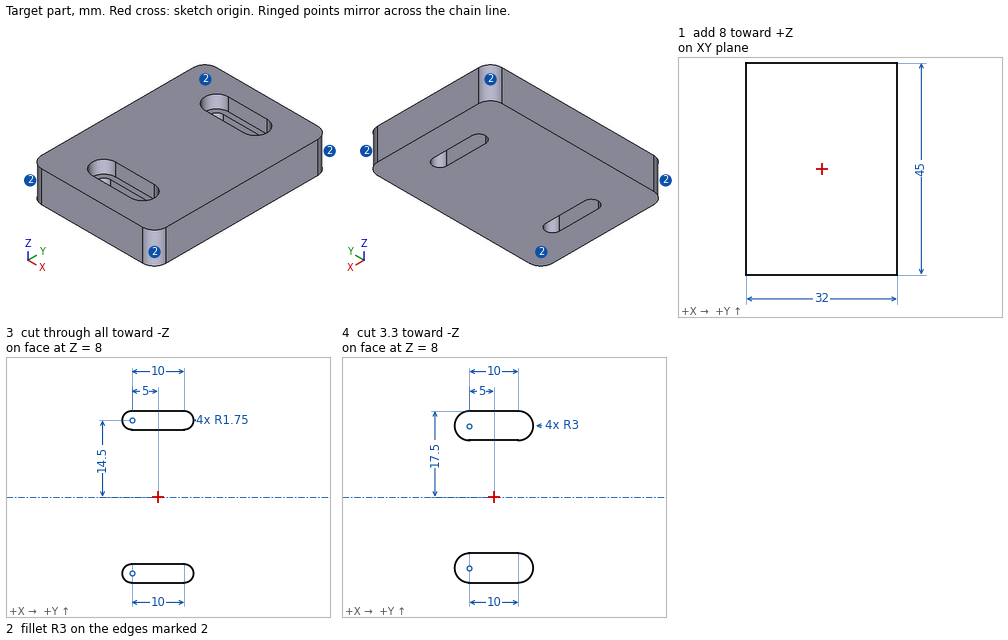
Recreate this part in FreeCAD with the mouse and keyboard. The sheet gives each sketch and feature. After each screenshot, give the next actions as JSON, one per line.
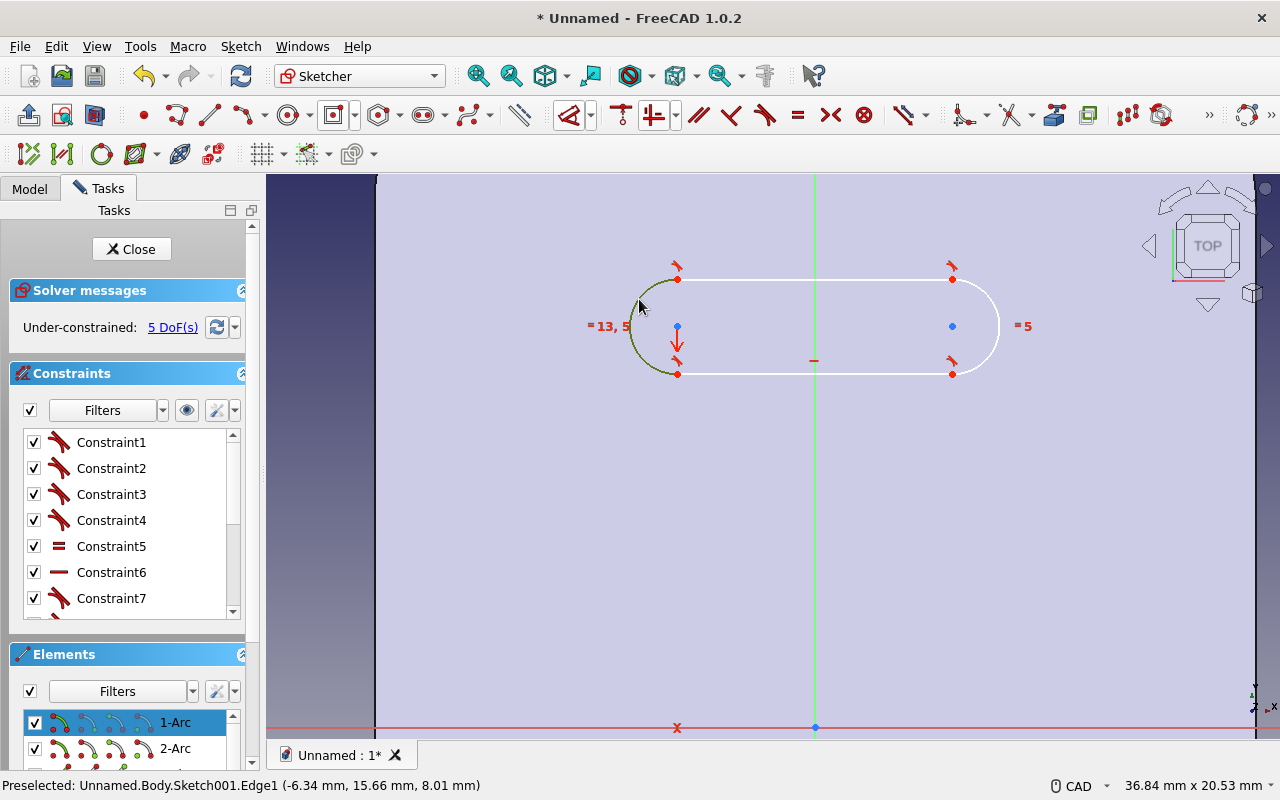
{"action": "left_click", "coordinate": [590, 116]}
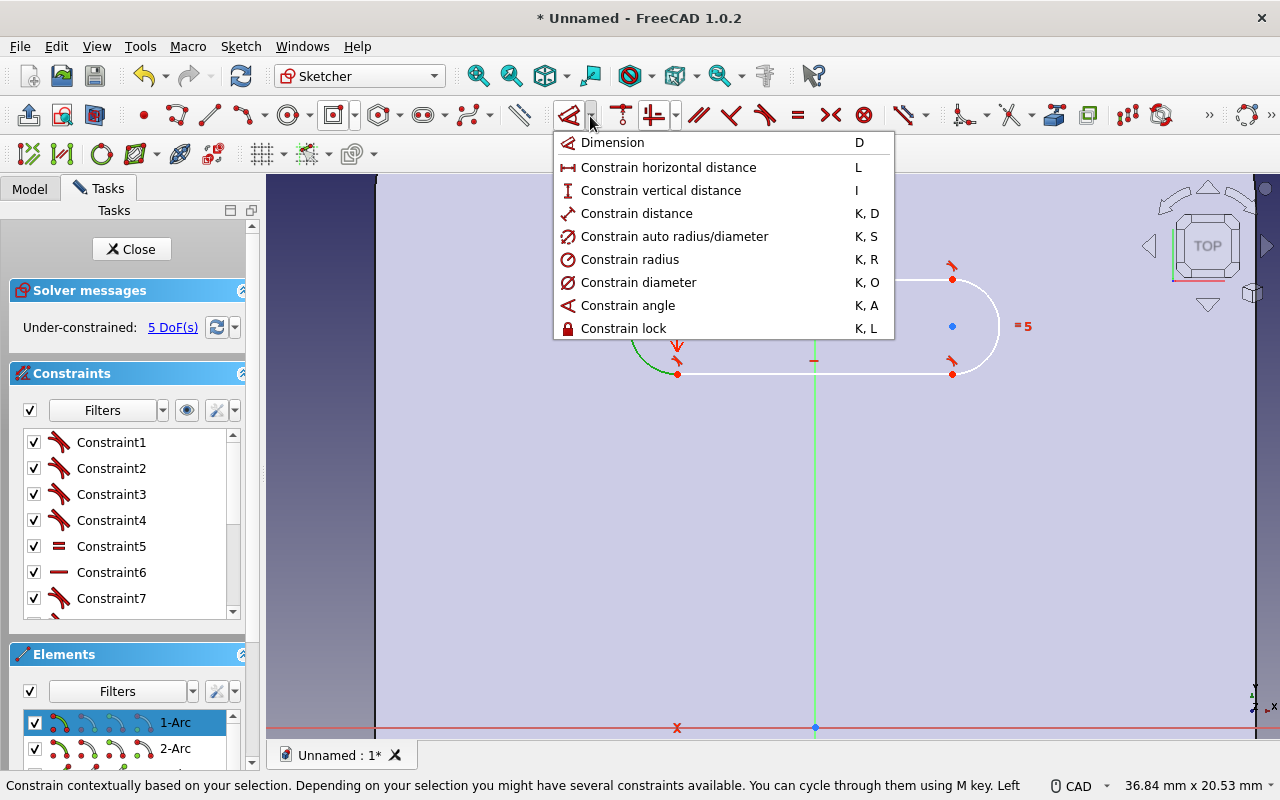
{"action": "left_click", "coordinate": [724, 260]}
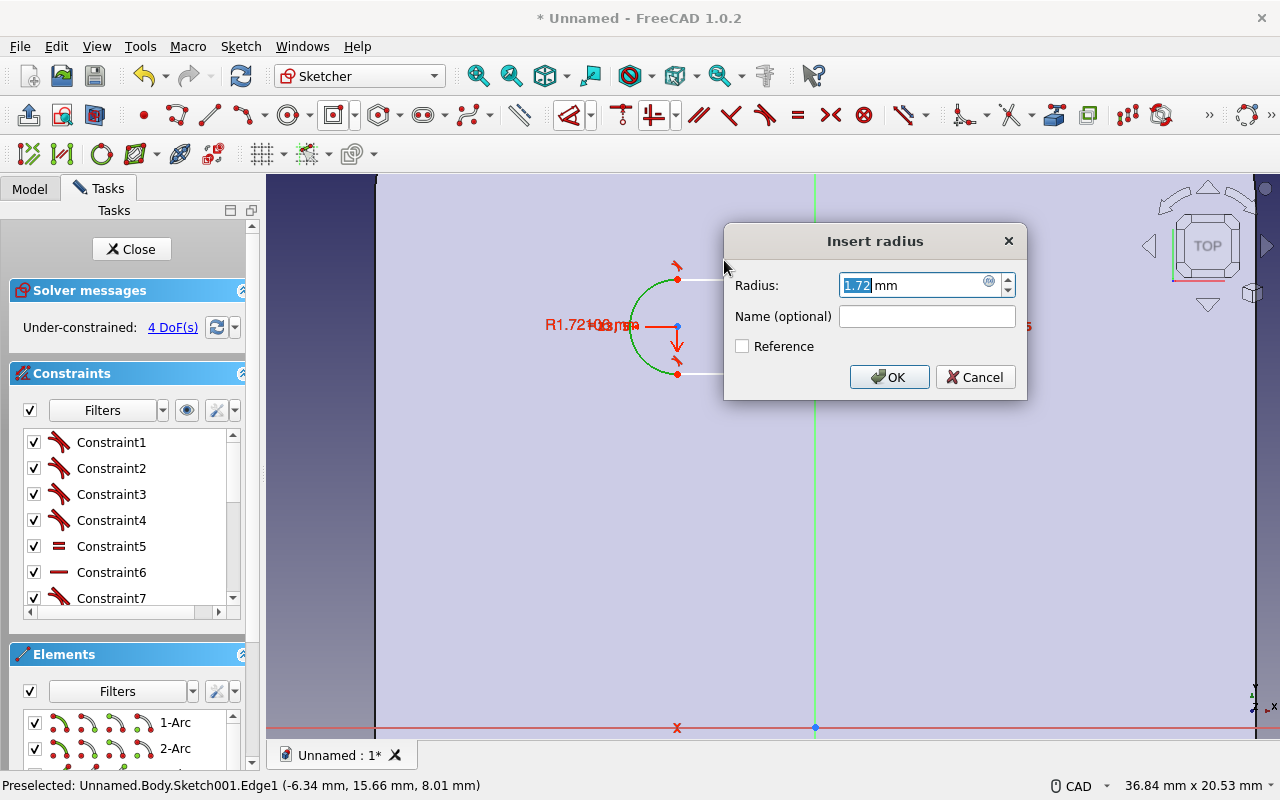
{"action": "type", "text": "1.75"}
{"action": "key", "text": "Return"}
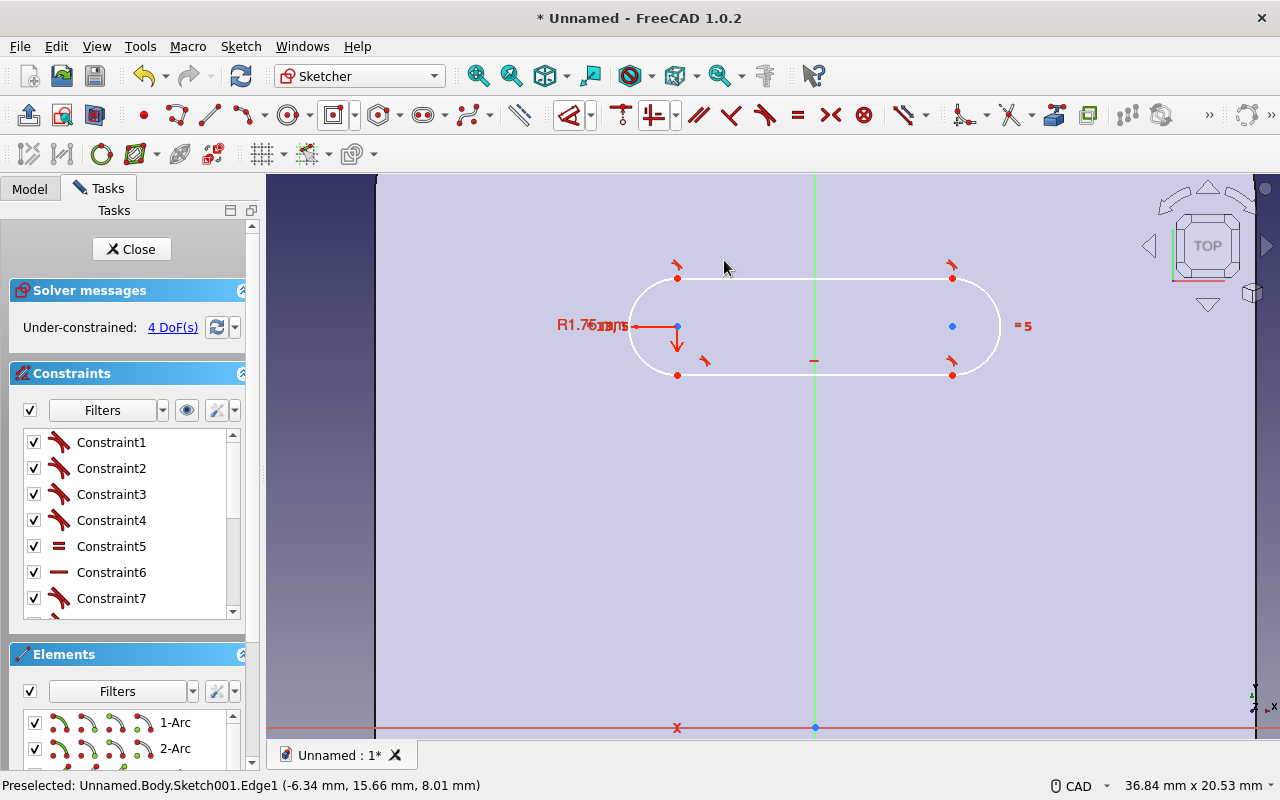
{"action": "left_click", "coordinate": [760, 279]}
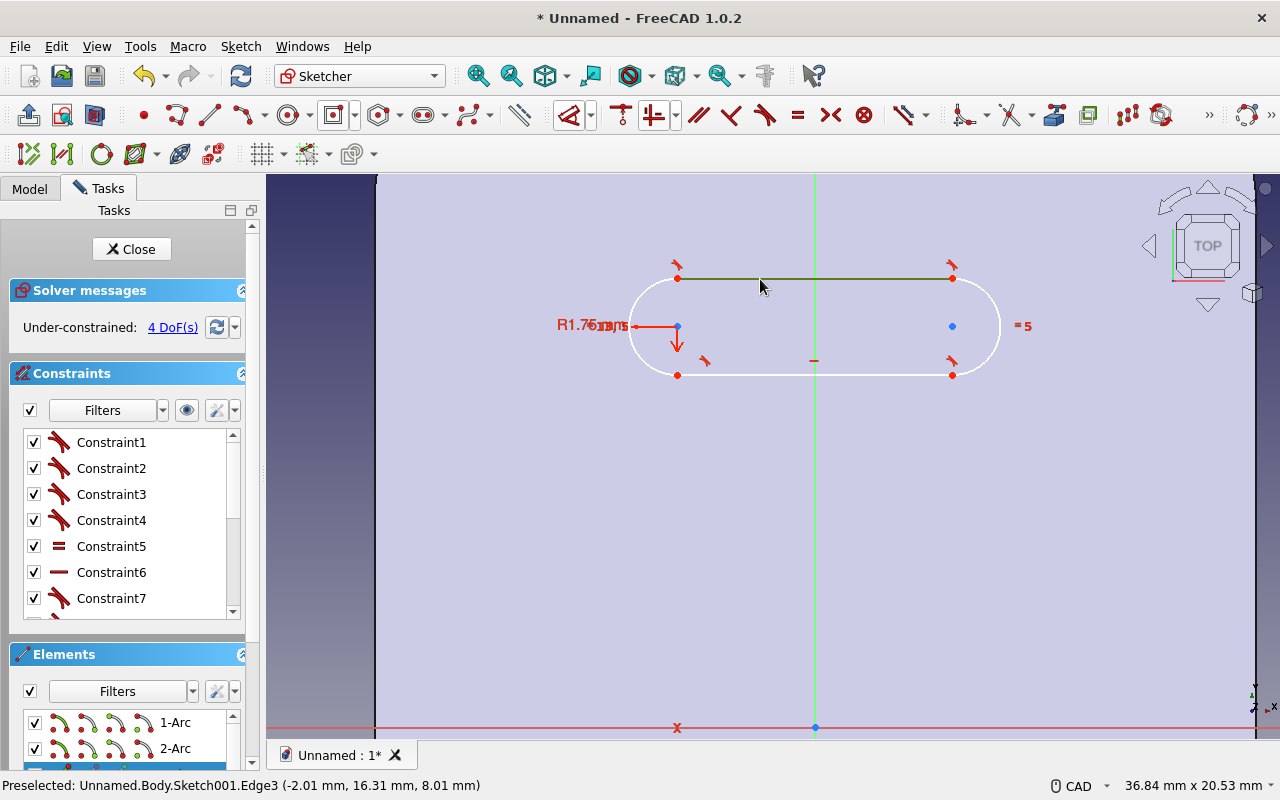
{"action": "left_click", "coordinate": [590, 116]}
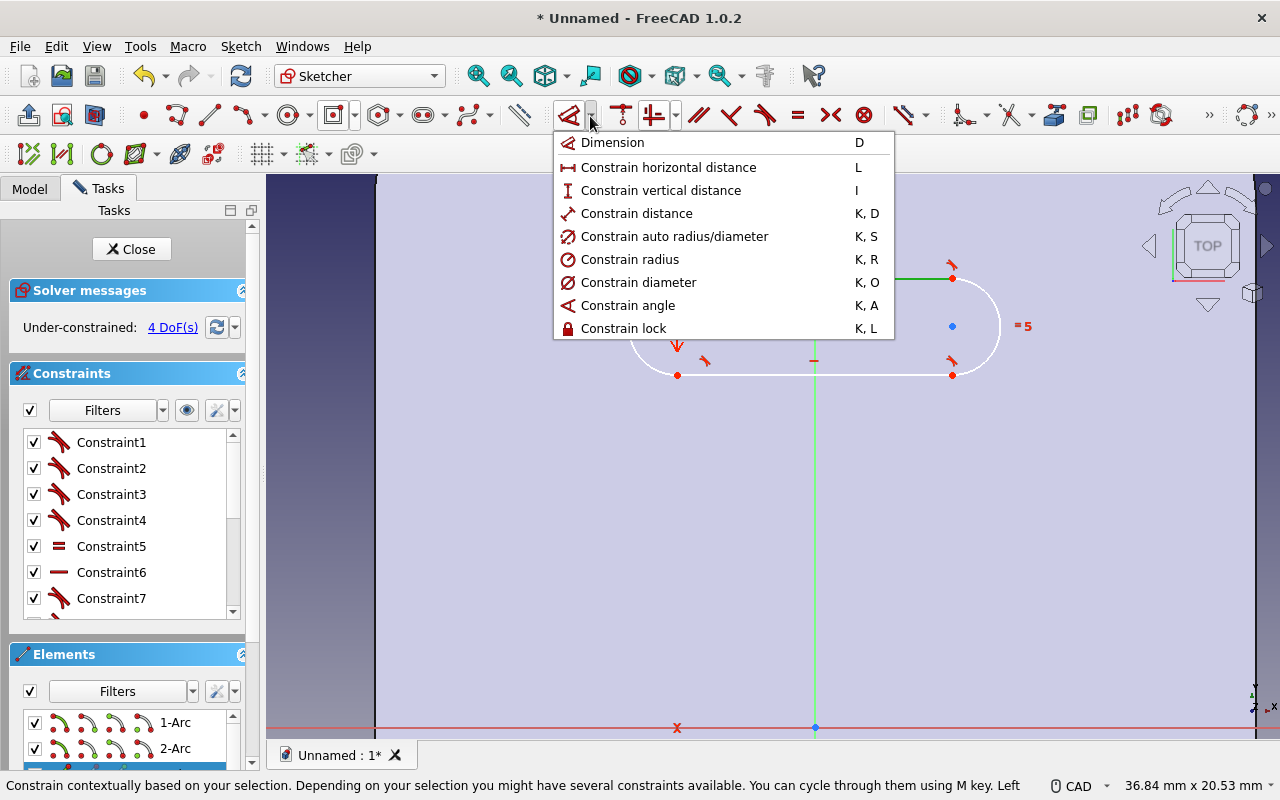
{"action": "left_click", "coordinate": [724, 168]}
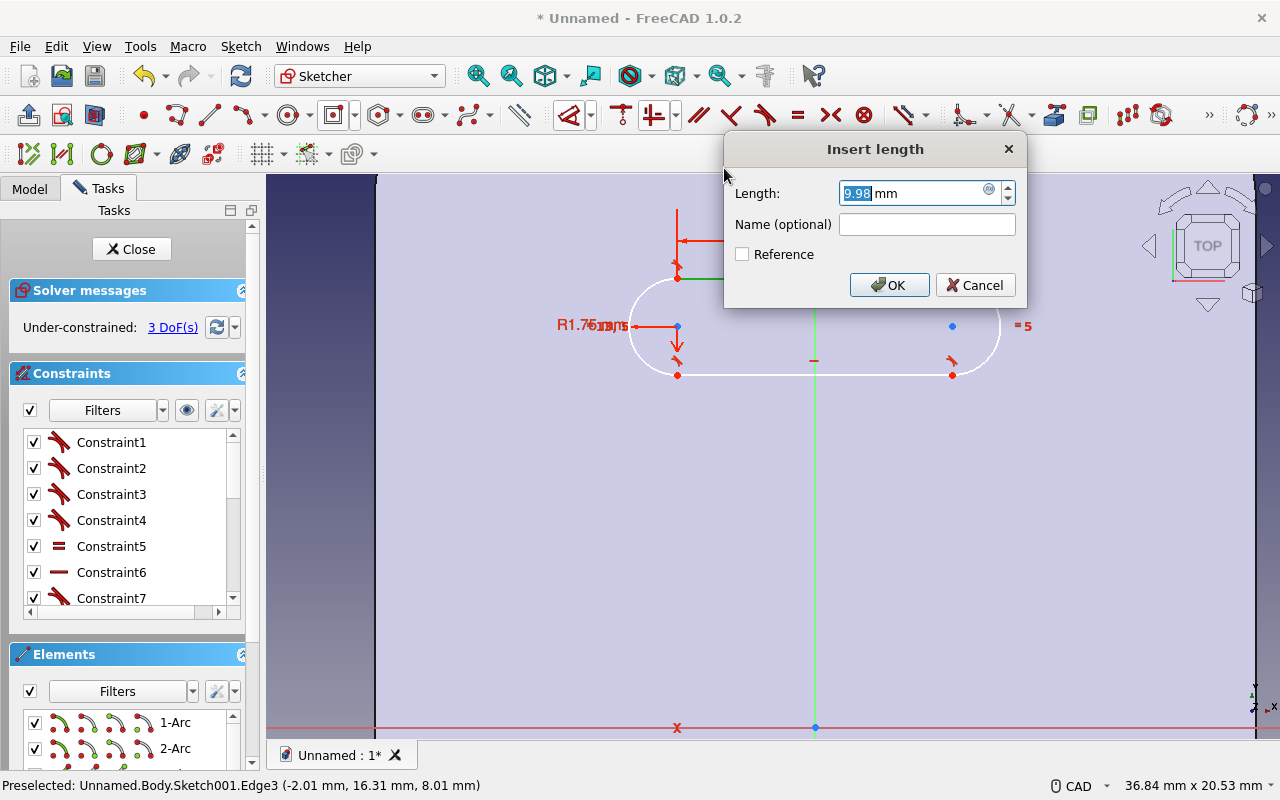
{"action": "type", "text": "10"}
{"action": "key", "text": "Return"}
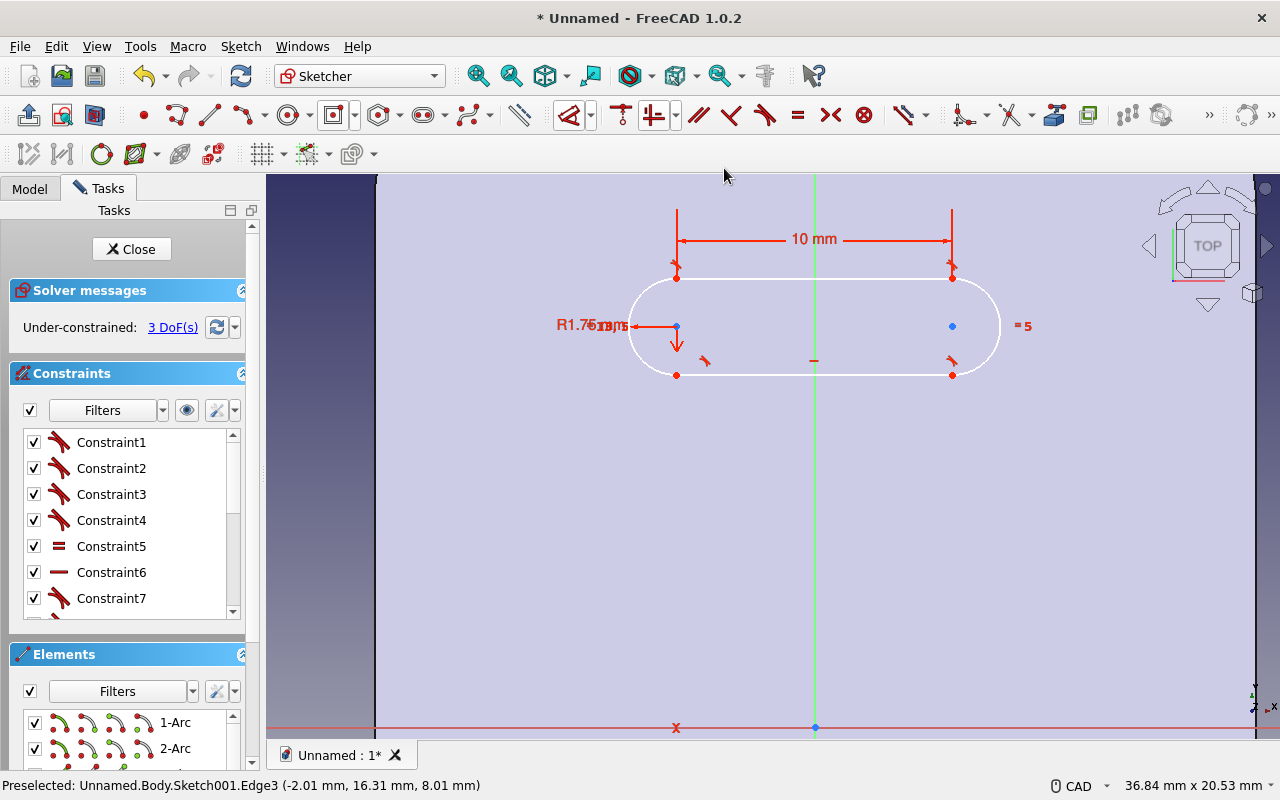
{"action": "scroll", "coordinate": [640, 299], "scroll_direction": "down", "scroll_amount": 5}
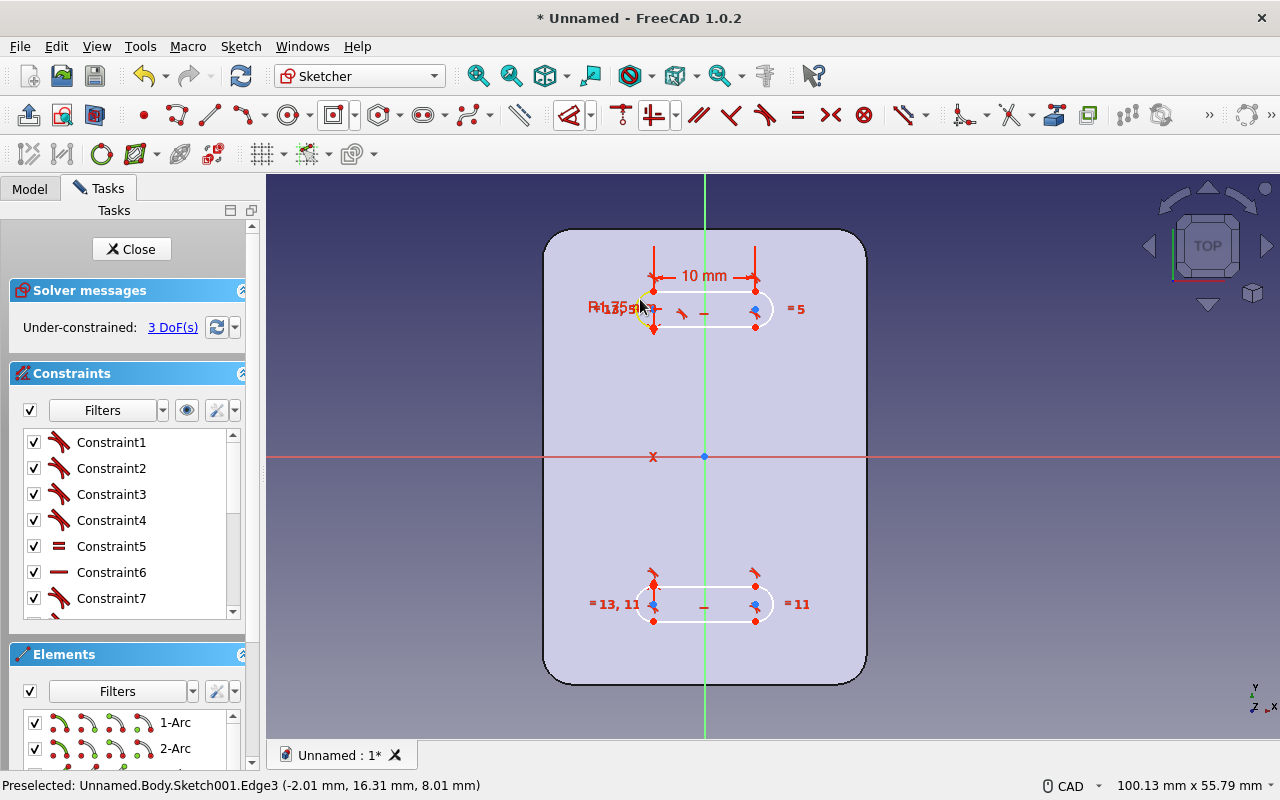
{"action": "left_click", "coordinate": [684, 587]}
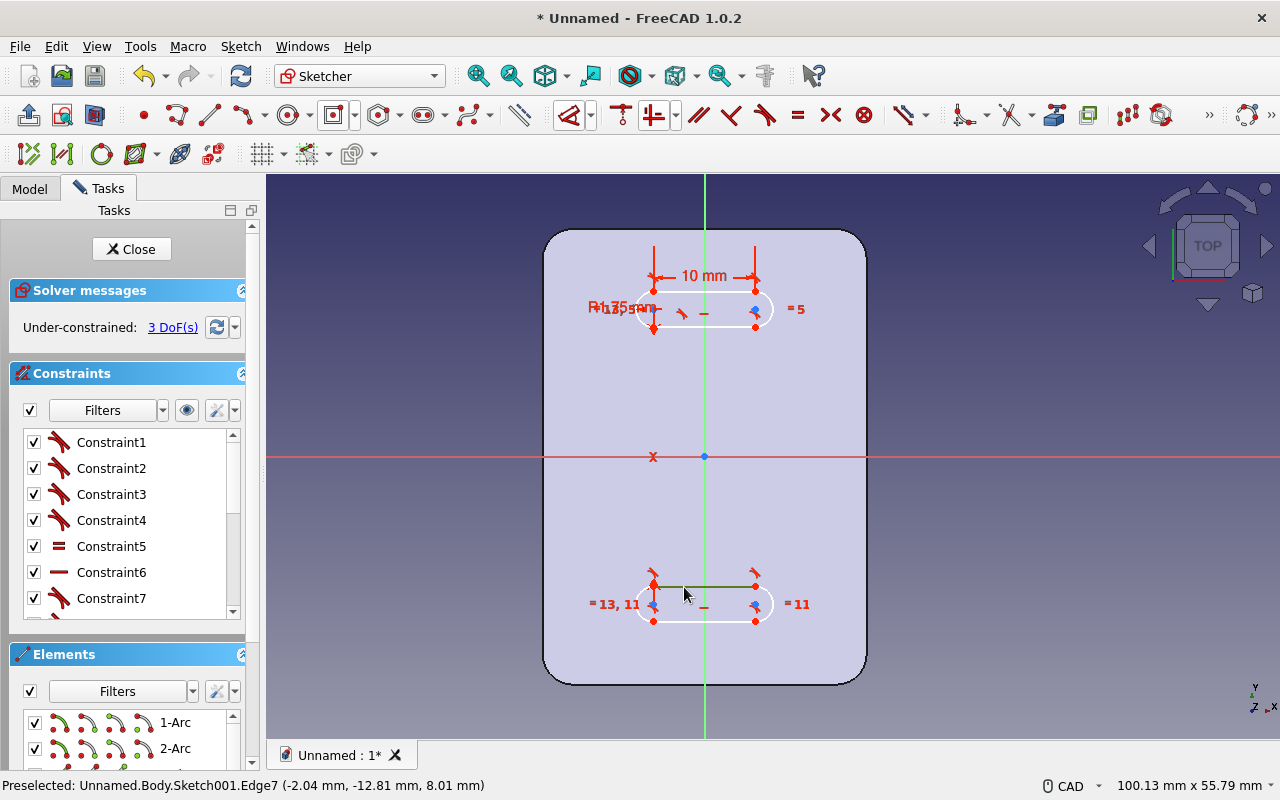
{"action": "left_click", "coordinate": [590, 116]}